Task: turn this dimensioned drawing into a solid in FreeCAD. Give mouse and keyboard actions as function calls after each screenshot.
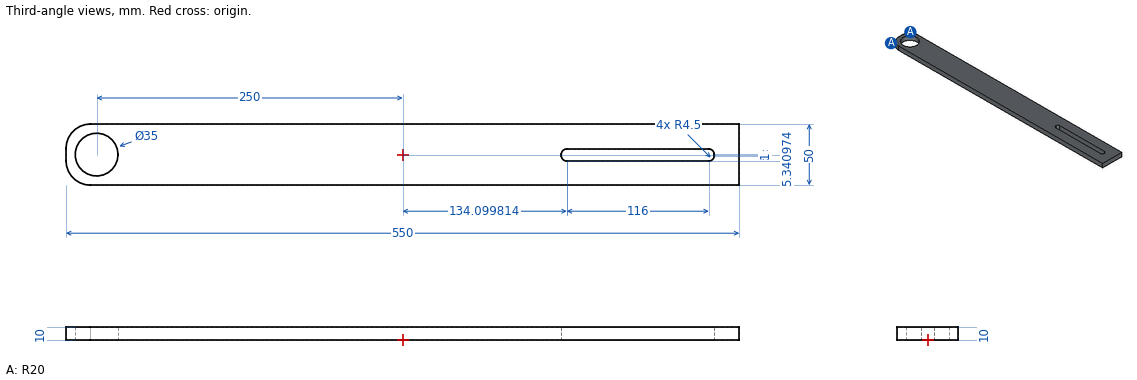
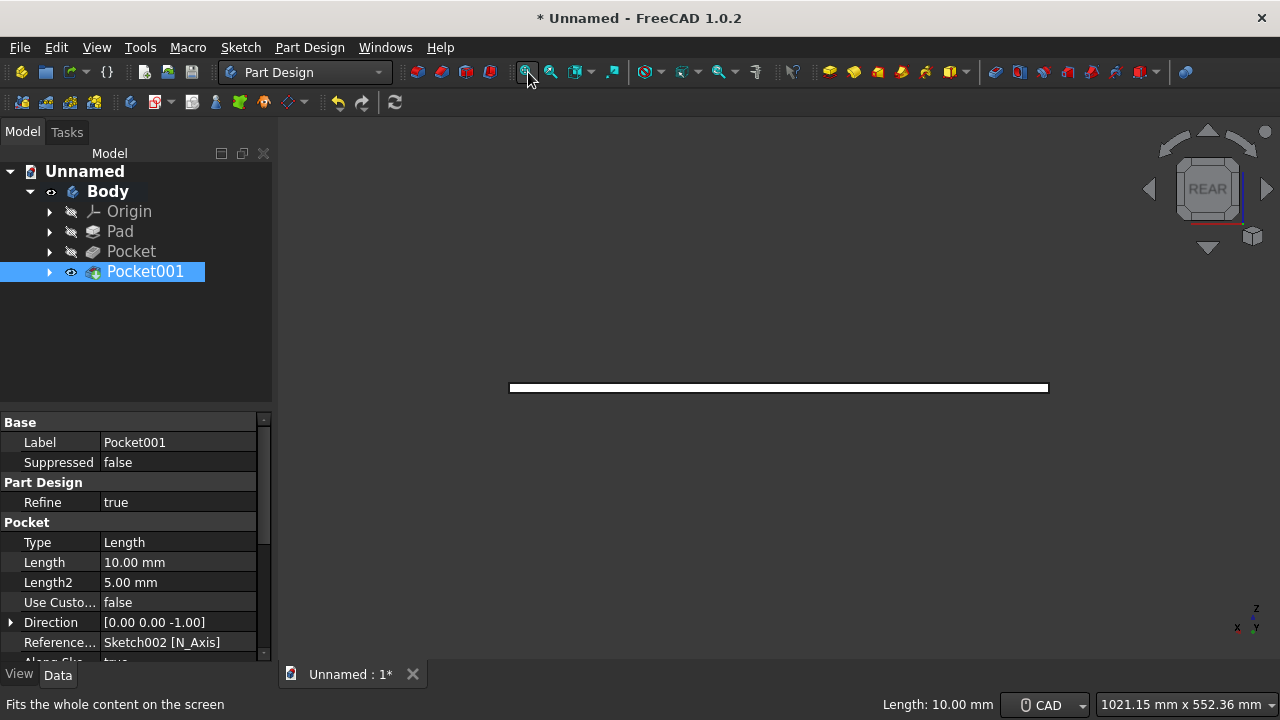
scroll(1049, 387, up, 8)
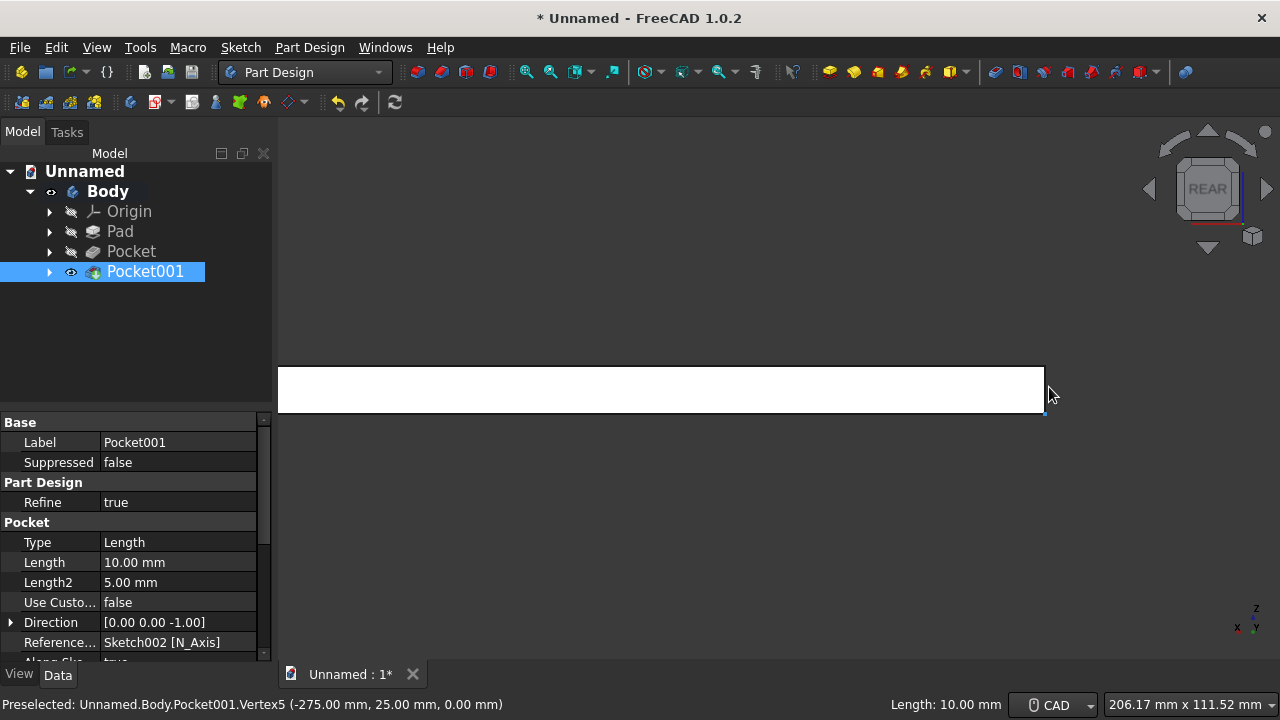
click(1045, 389, ctrl)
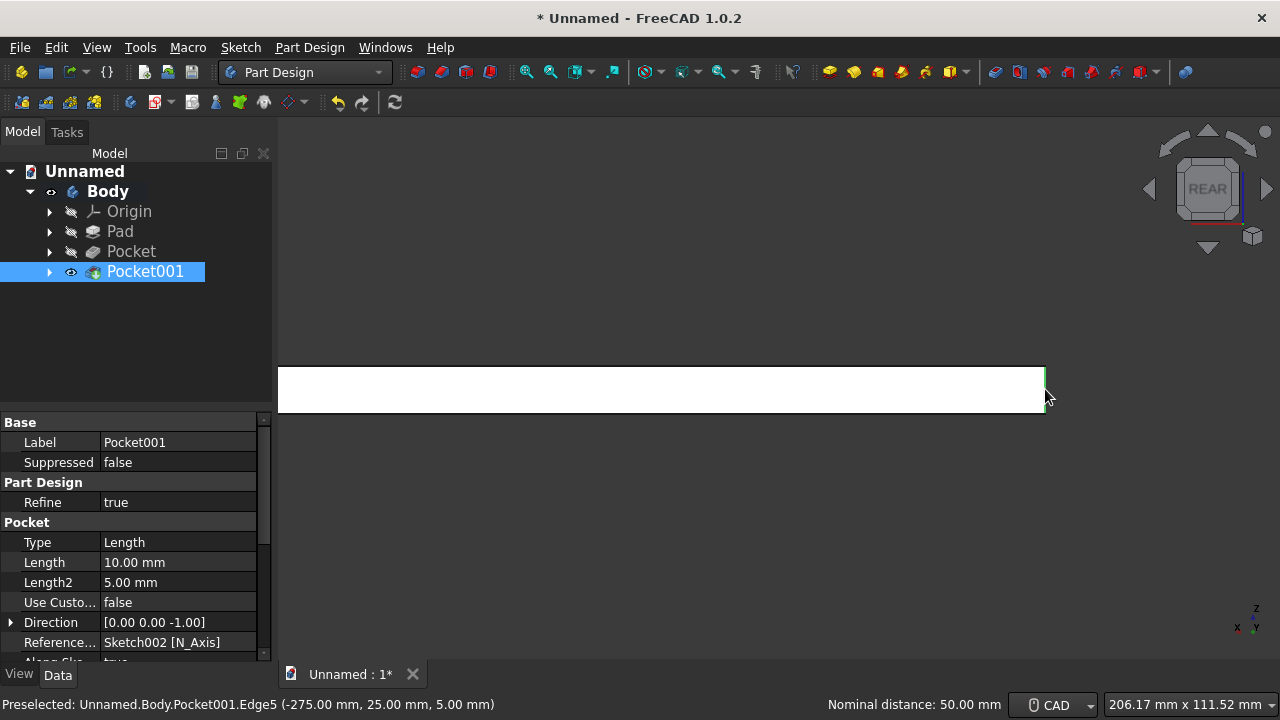
click(418, 72)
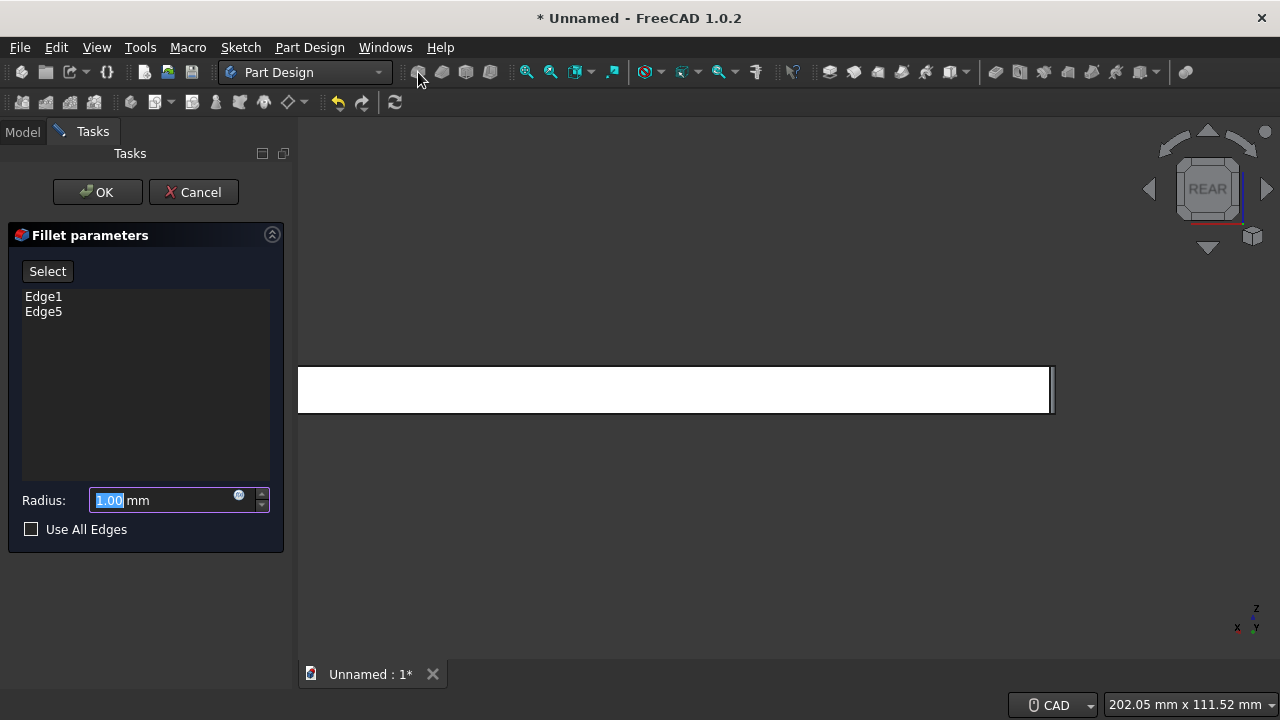
text(20)
key(Tab)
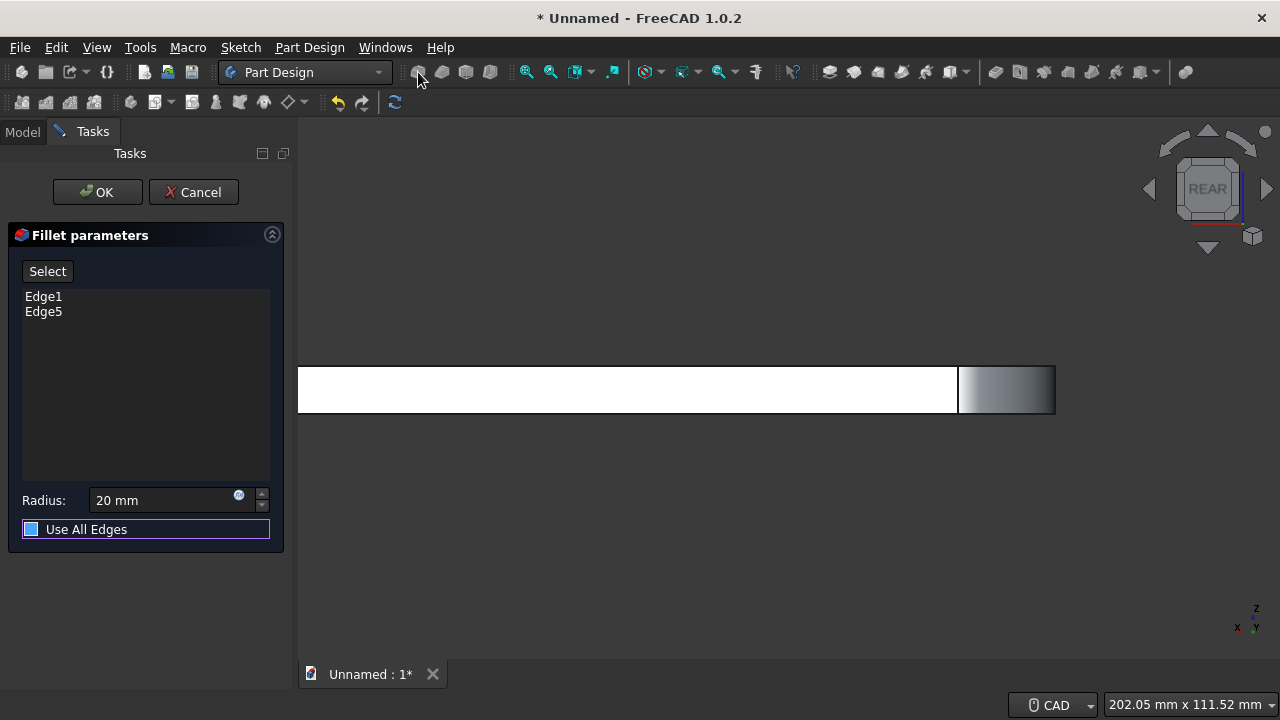
click(98, 192)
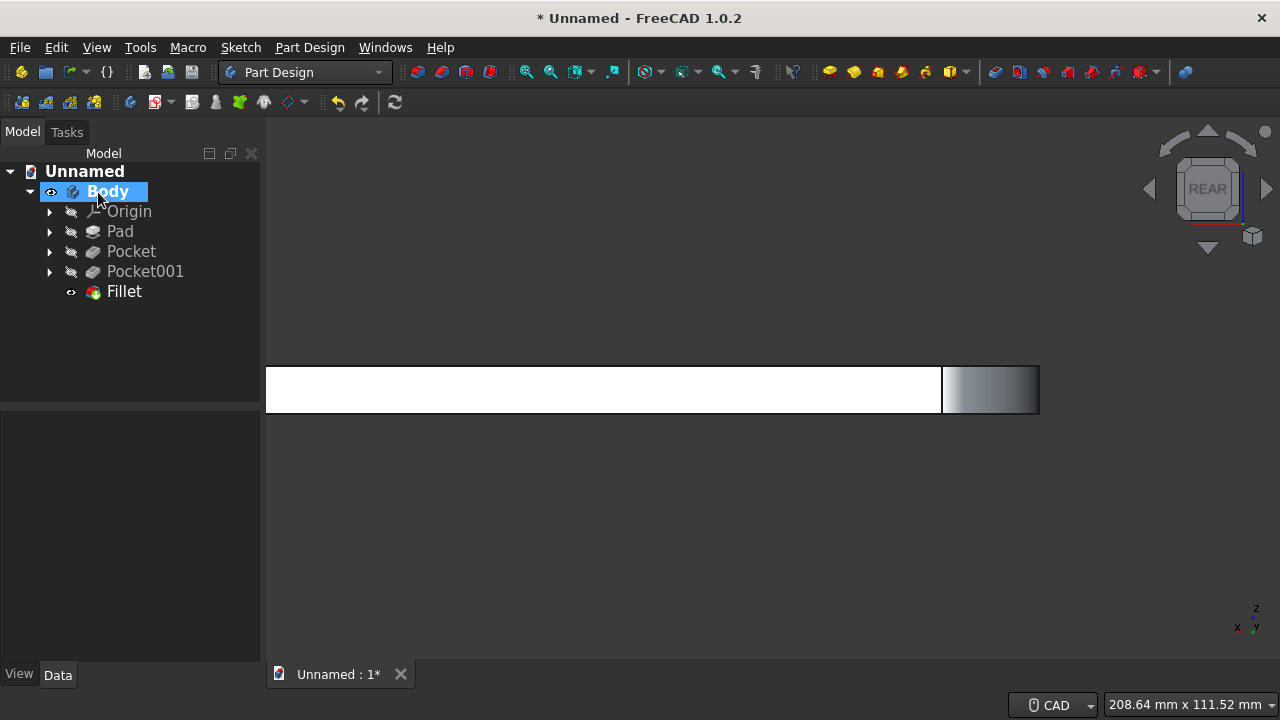
key(0)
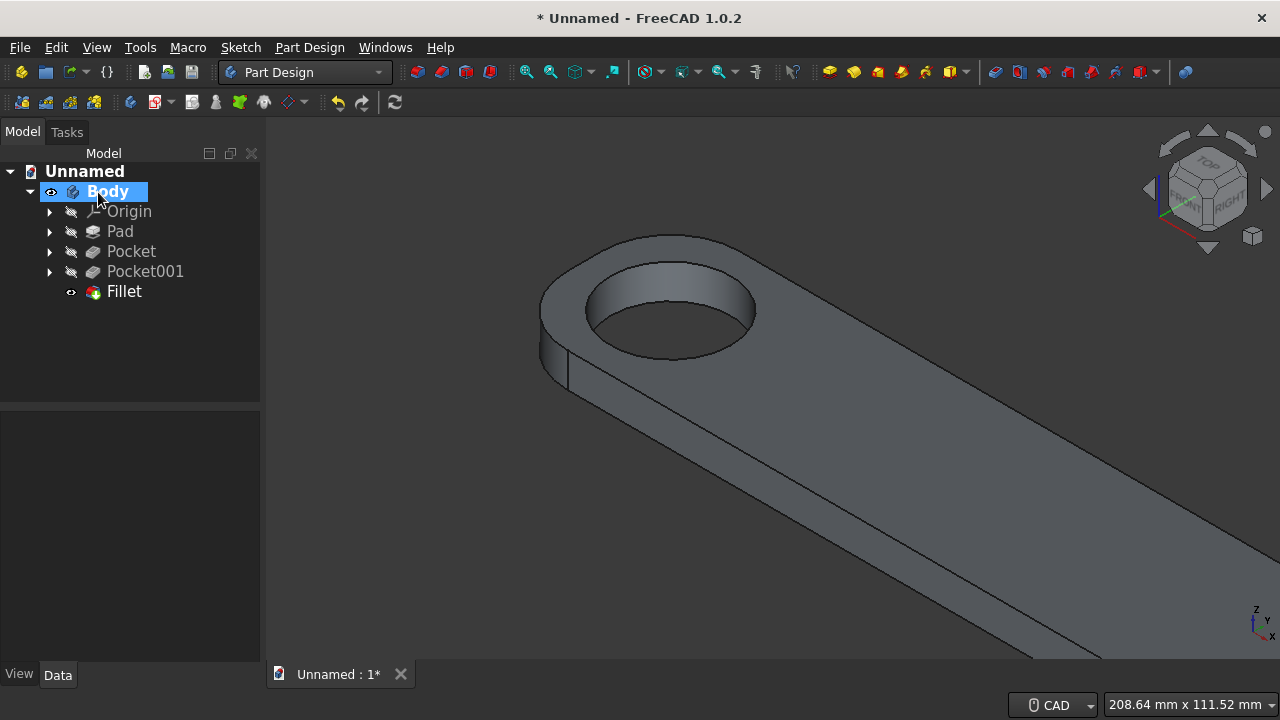
click(528, 72)